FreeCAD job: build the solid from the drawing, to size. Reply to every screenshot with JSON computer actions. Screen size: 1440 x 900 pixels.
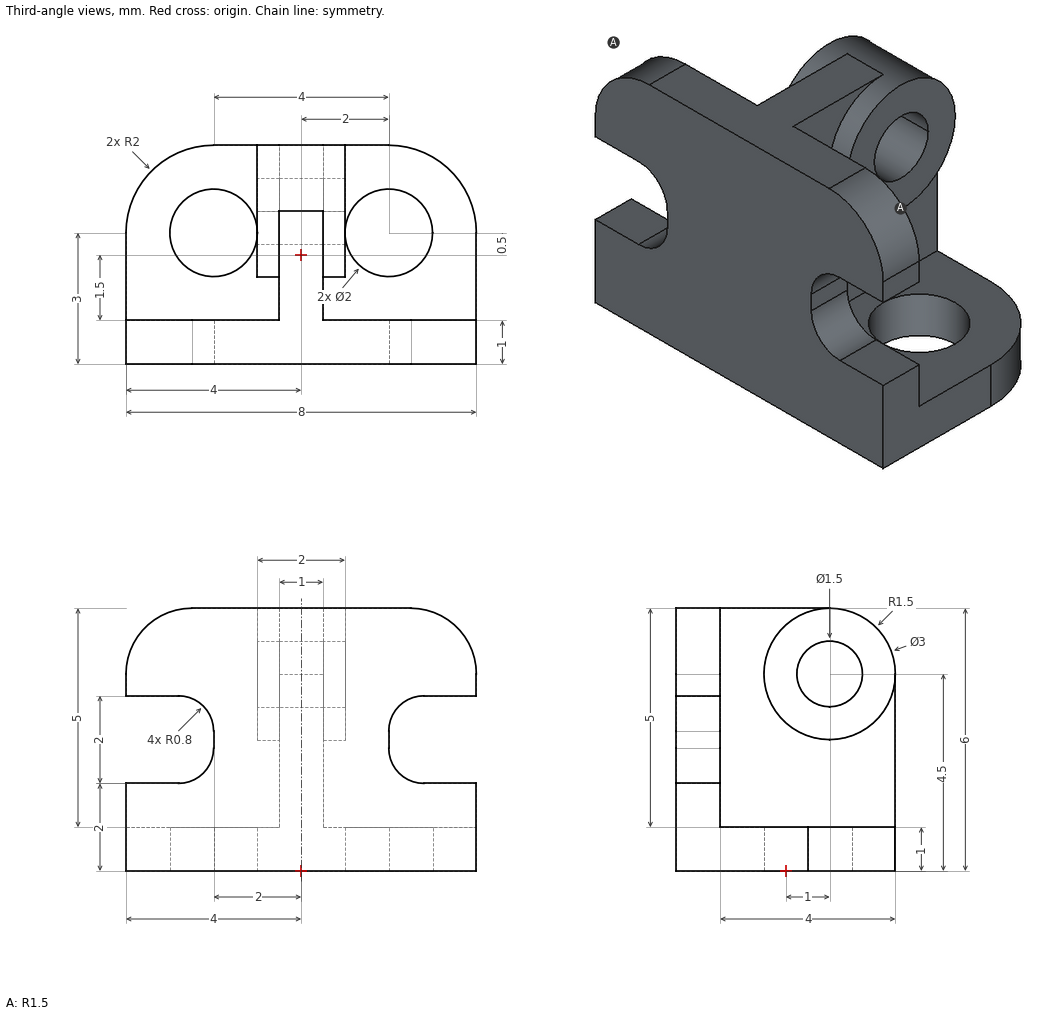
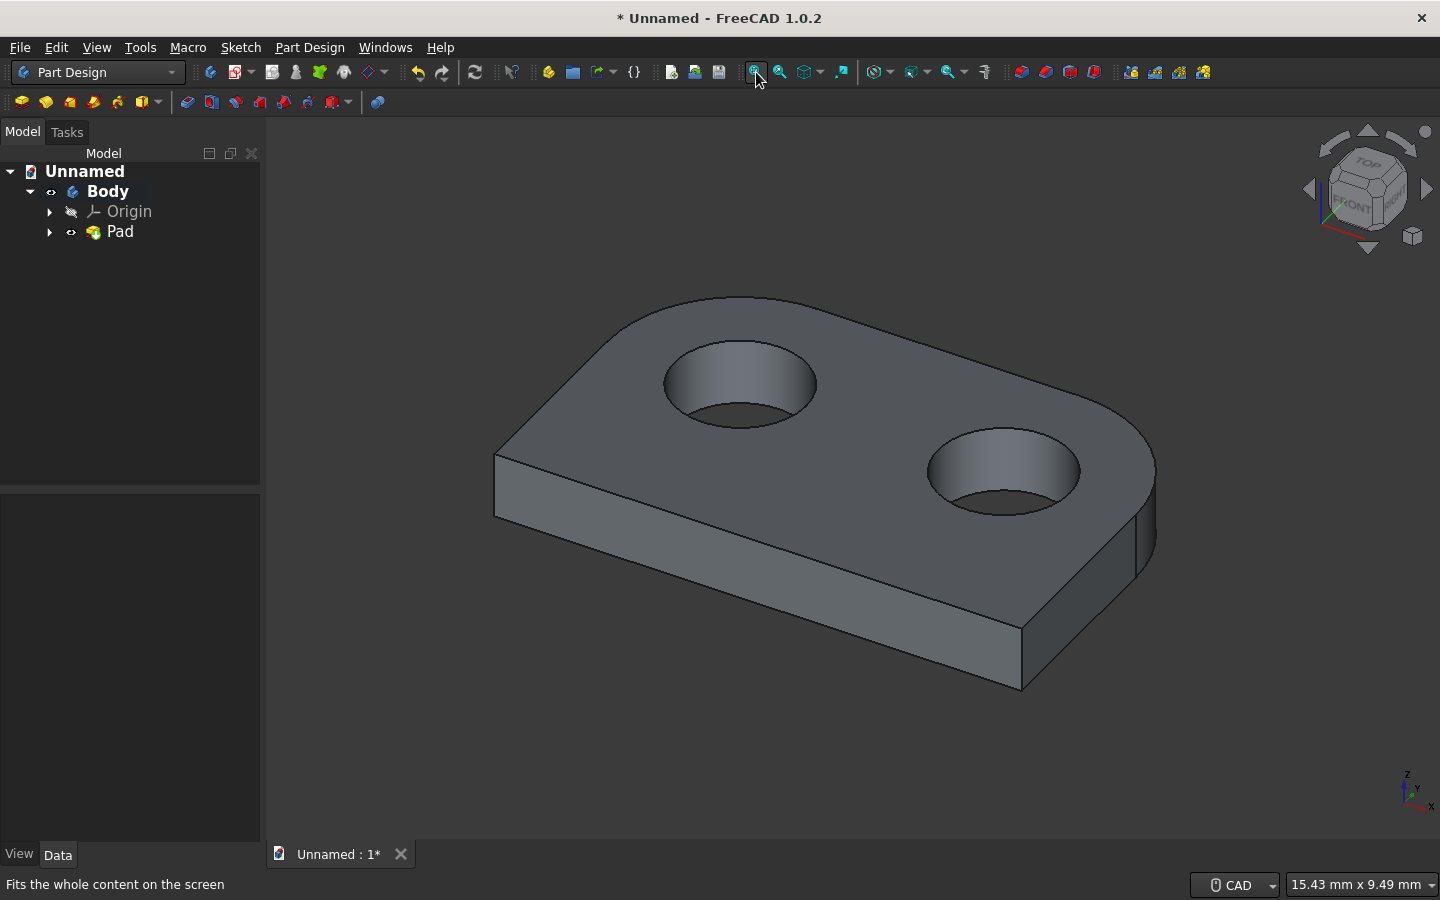
{"action": "left_click", "coordinate": [826, 473]}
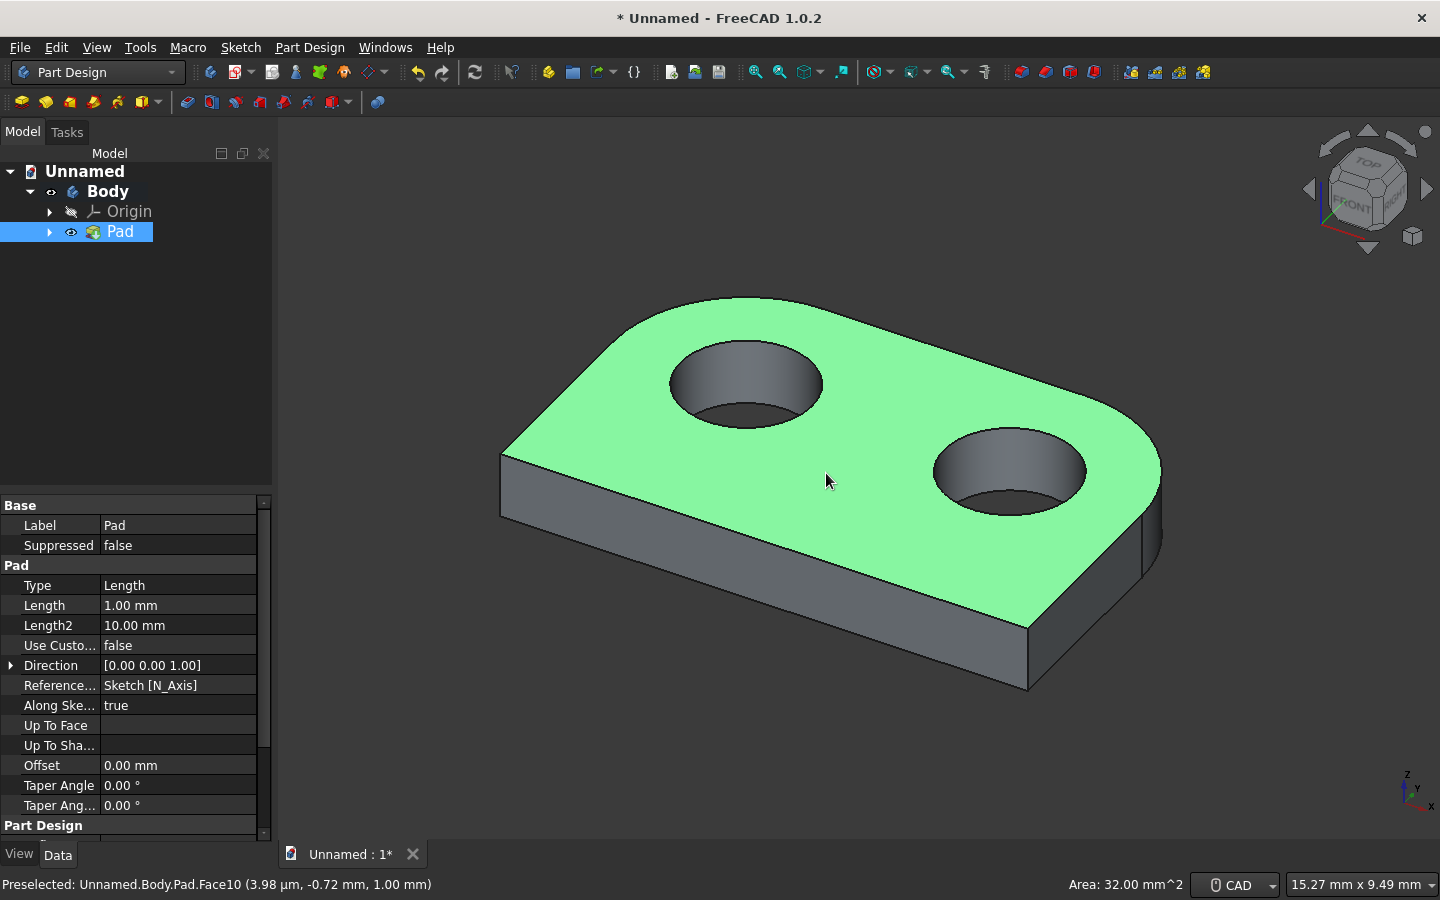
{"action": "left_click", "coordinate": [236, 72]}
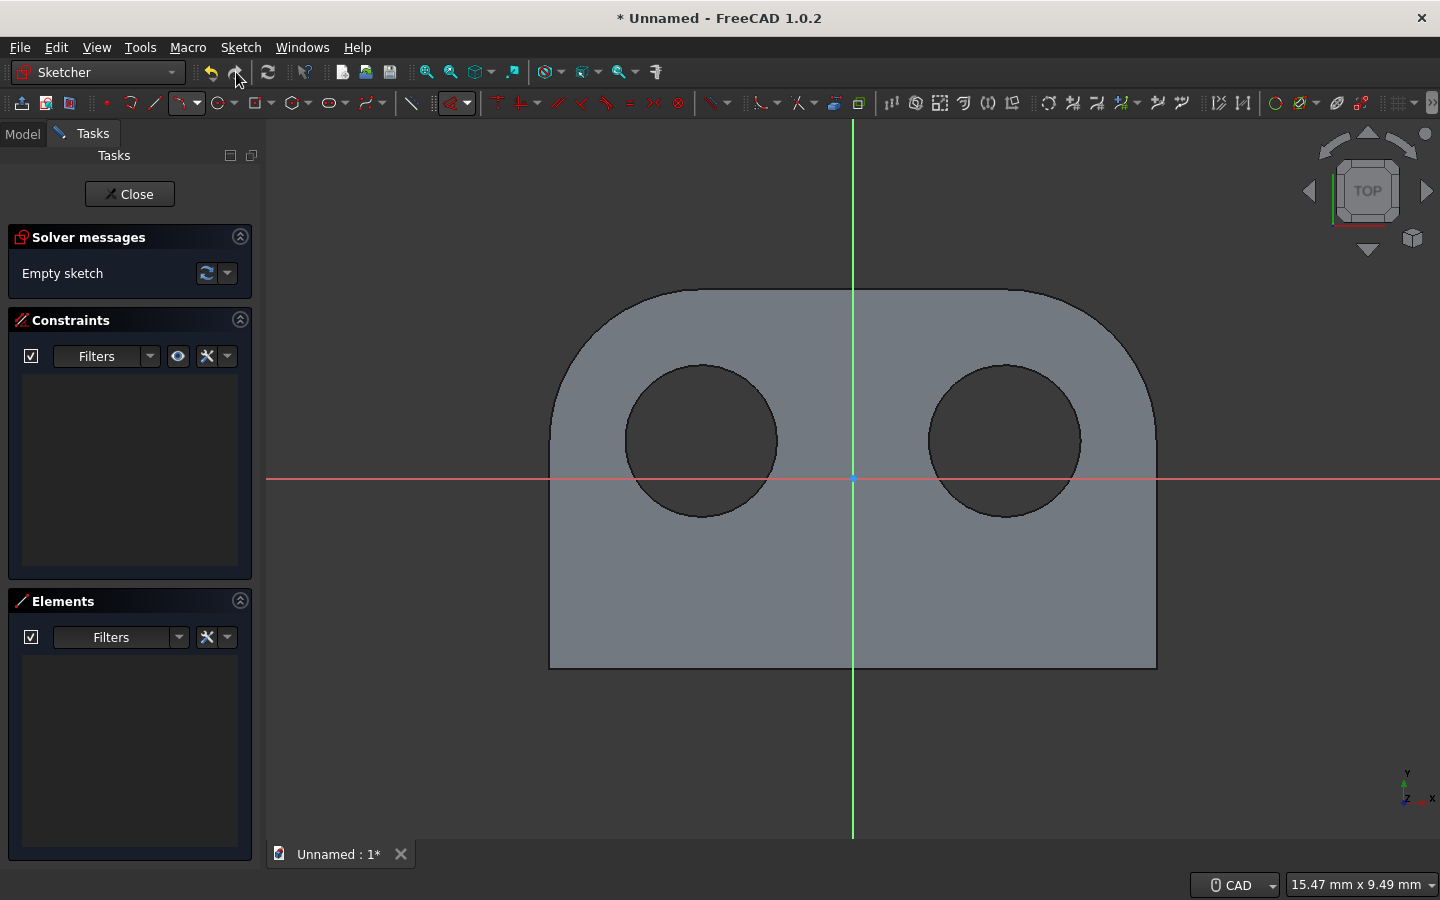
{"action": "key", "text": "g r"}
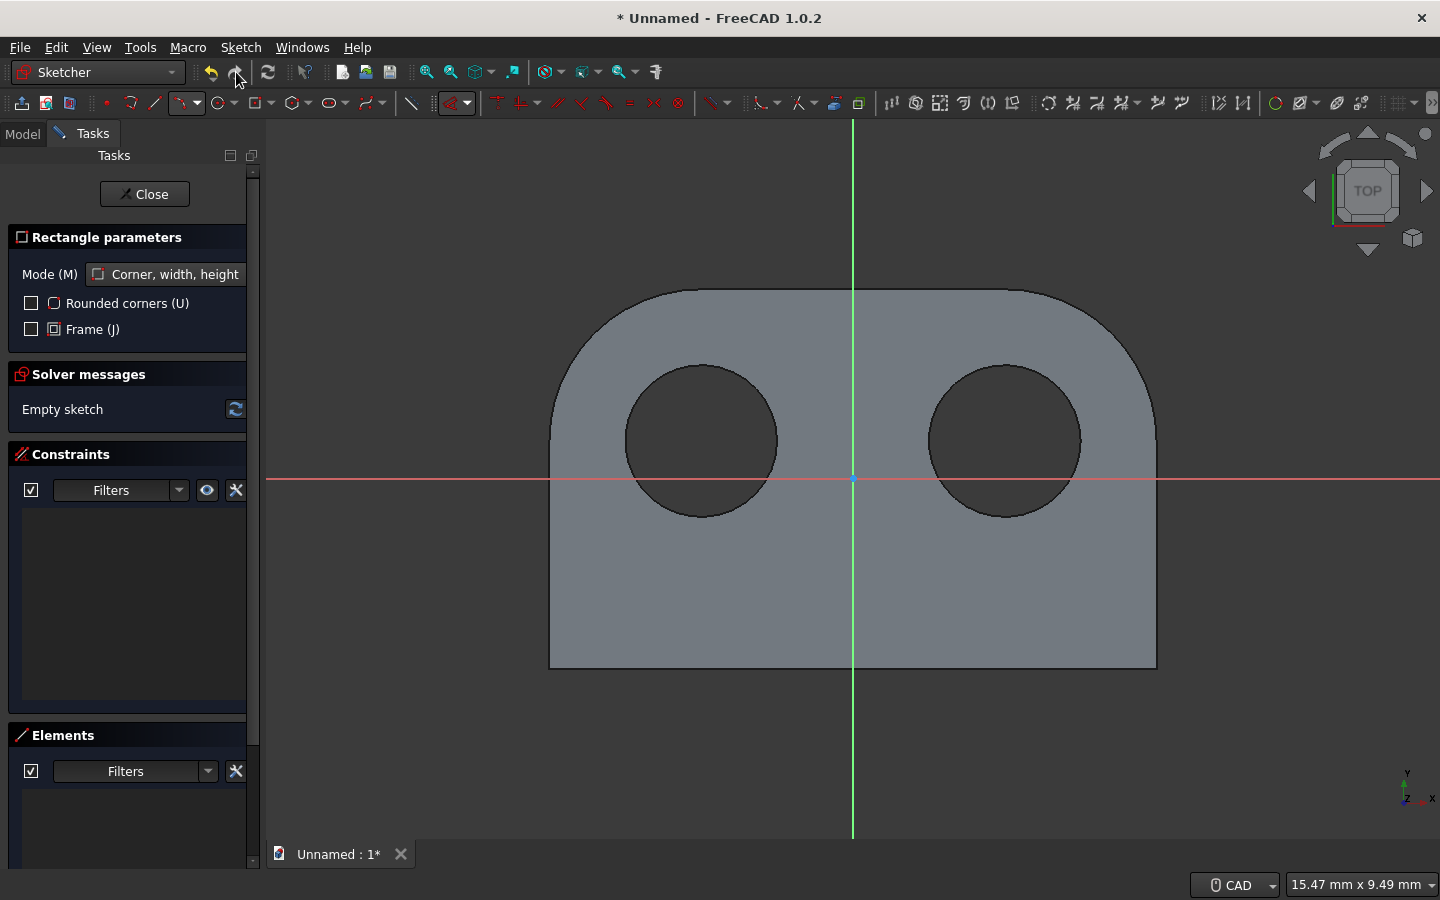
{"action": "left_click", "coordinate": [549, 593]}
{"action": "mouse_move", "coordinate": [1157, 669]}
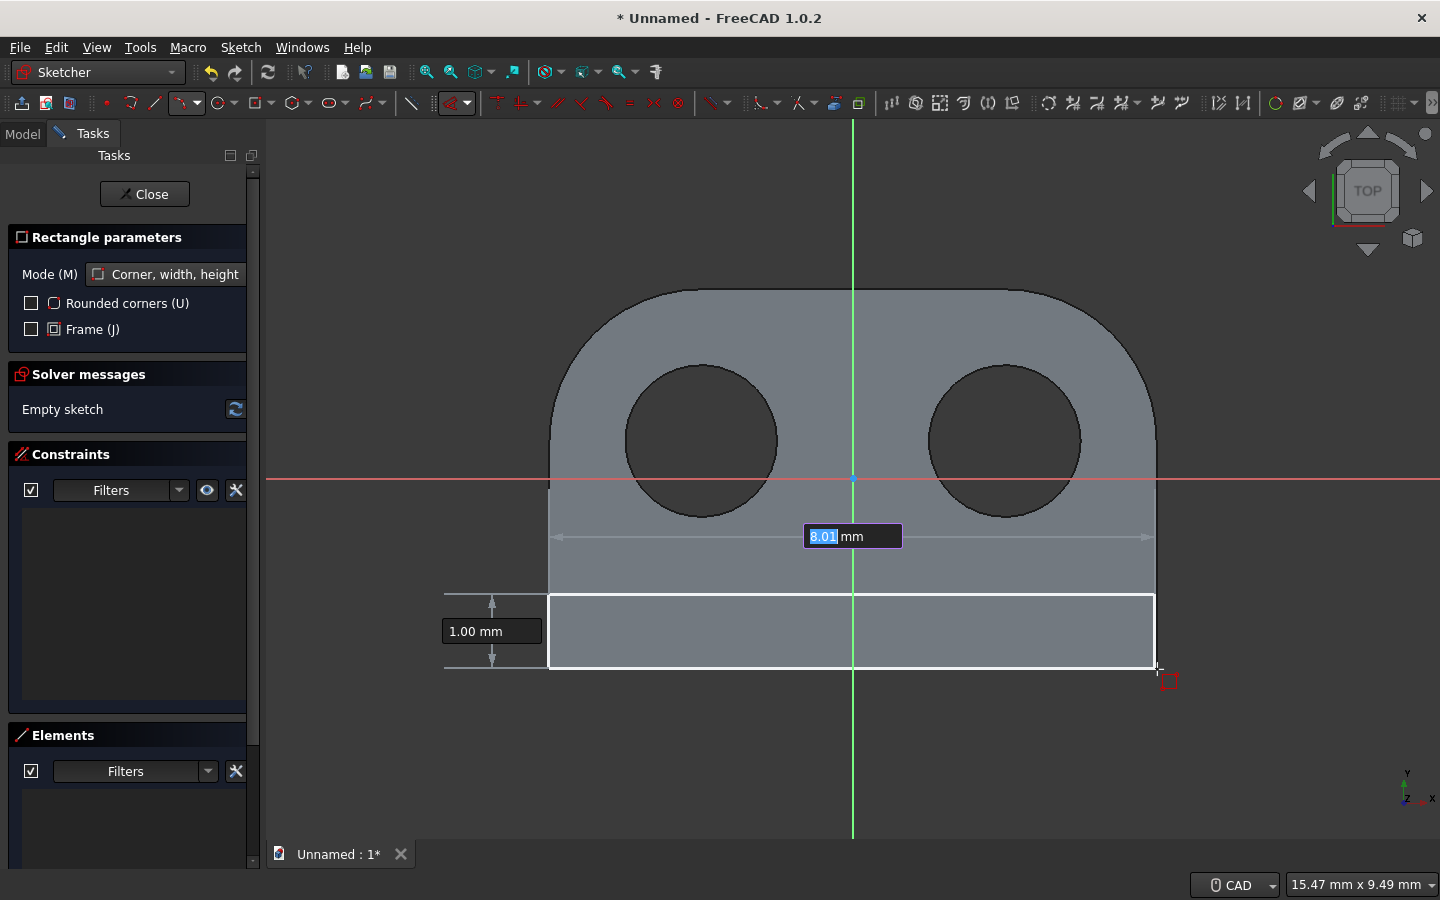
{"action": "type", "text": "8"}
{"action": "key", "text": "Tab"}
{"action": "type", "text": "1"}
{"action": "key", "text": "Return"}
{"action": "key", "text": "Escape"}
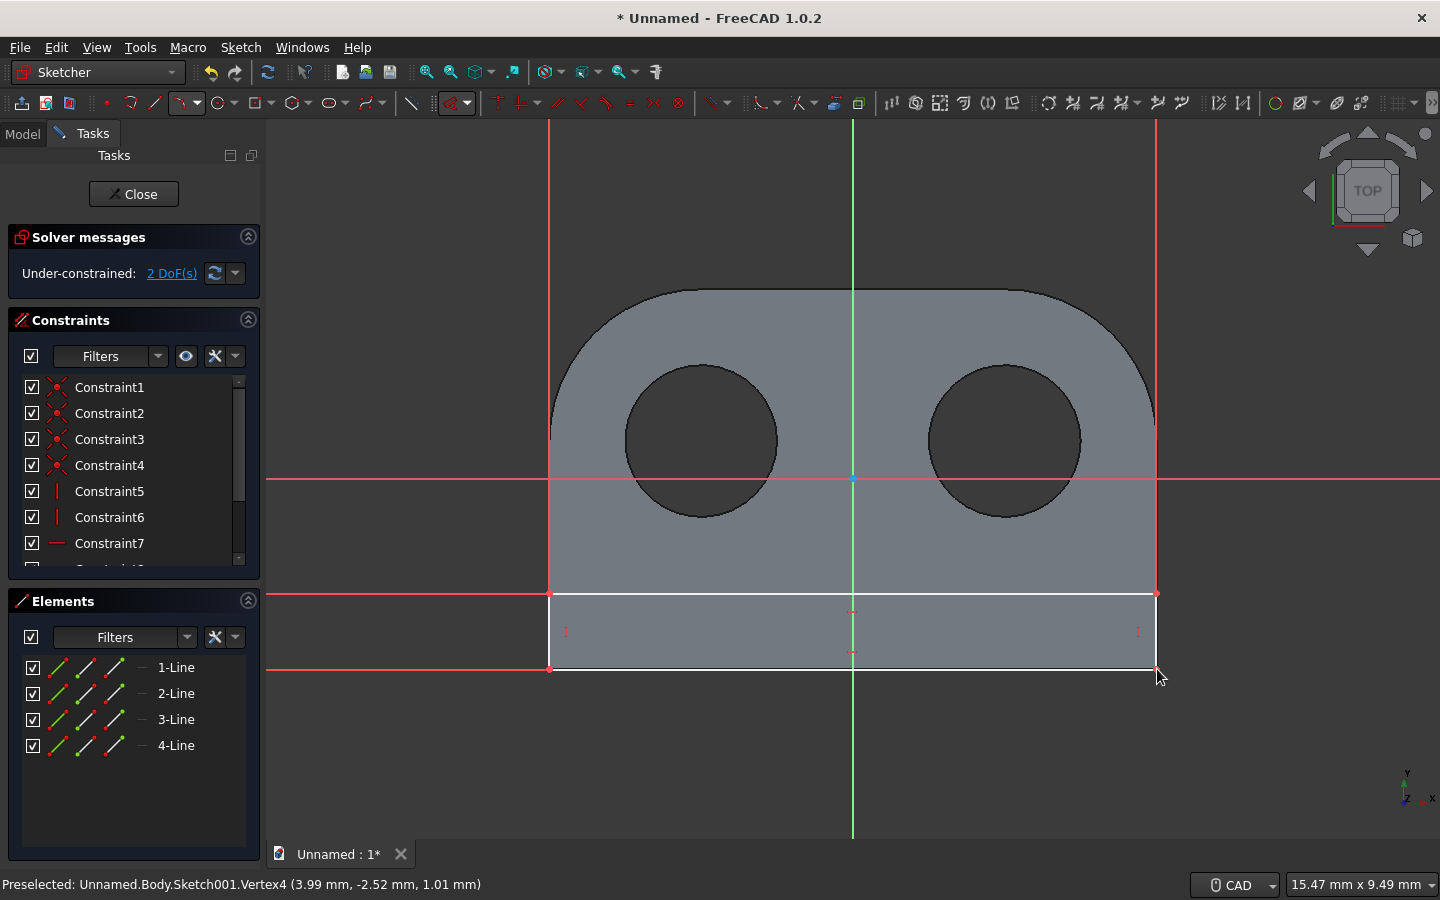
{"action": "left_click", "coordinate": [549, 594]}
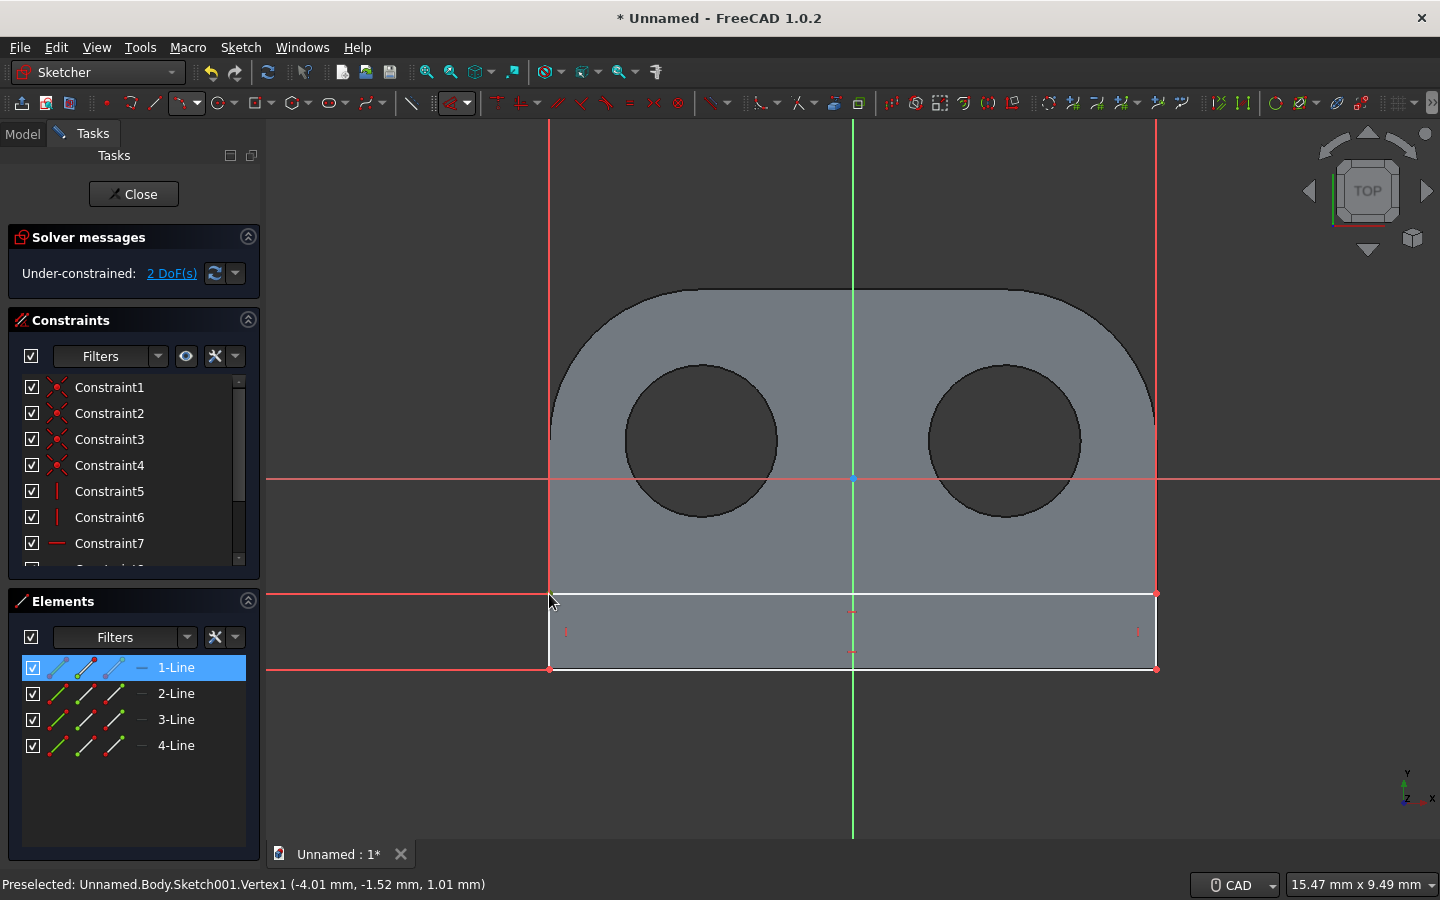
{"action": "left_click", "coordinate": [470, 104]}